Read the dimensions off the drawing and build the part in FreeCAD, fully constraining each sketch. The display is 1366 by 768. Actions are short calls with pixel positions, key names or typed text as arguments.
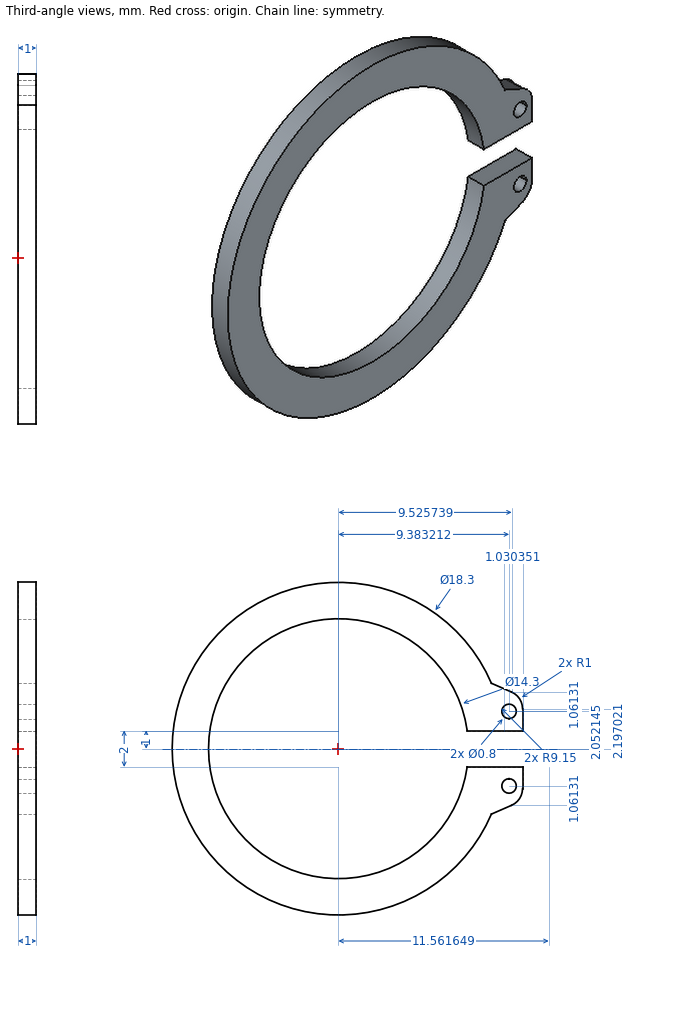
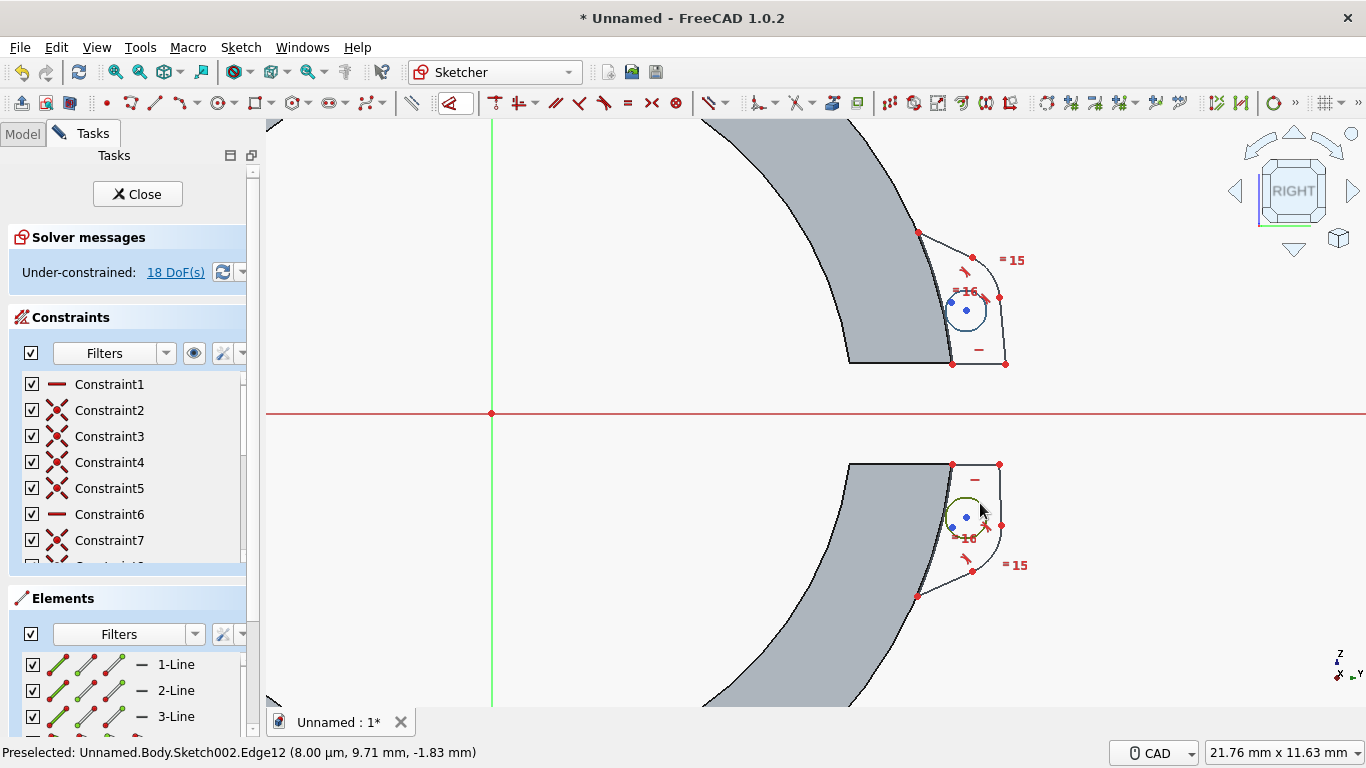
click(628, 104)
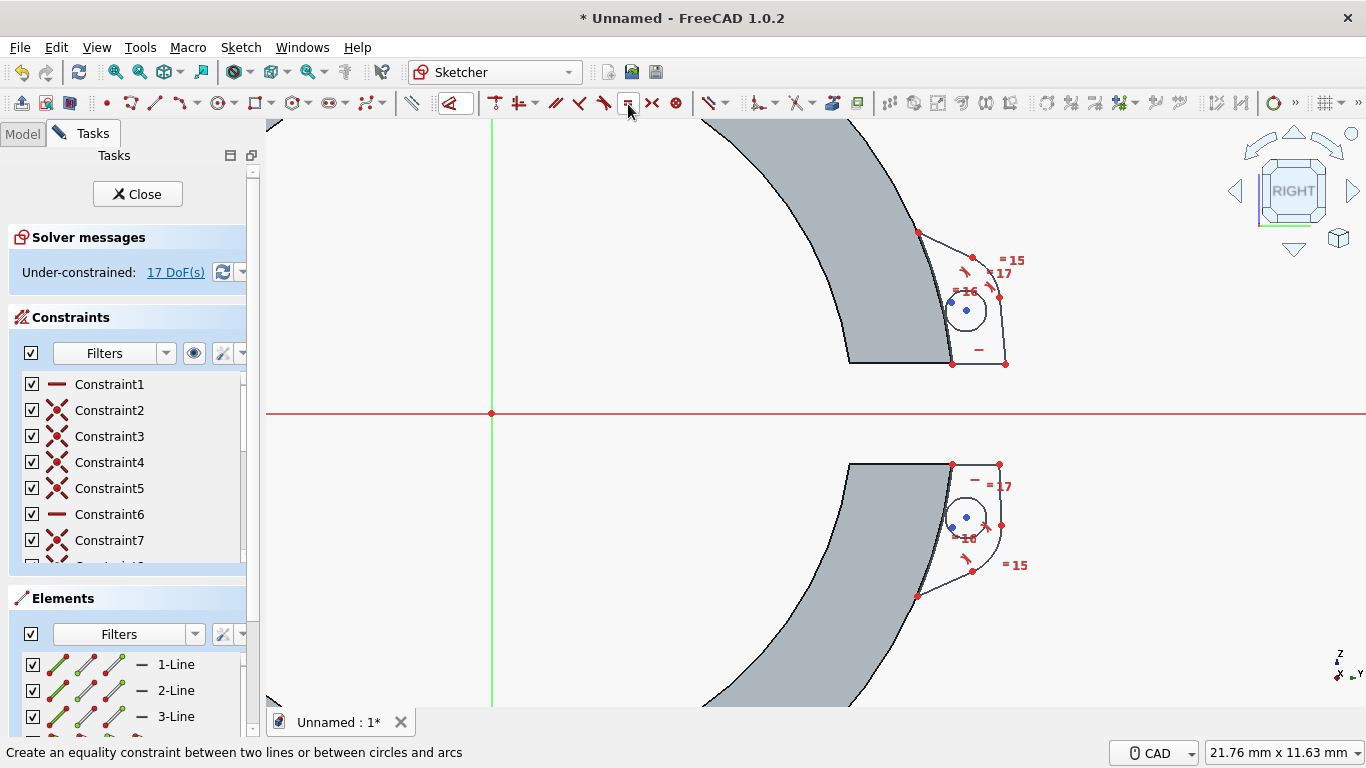
click(951, 302)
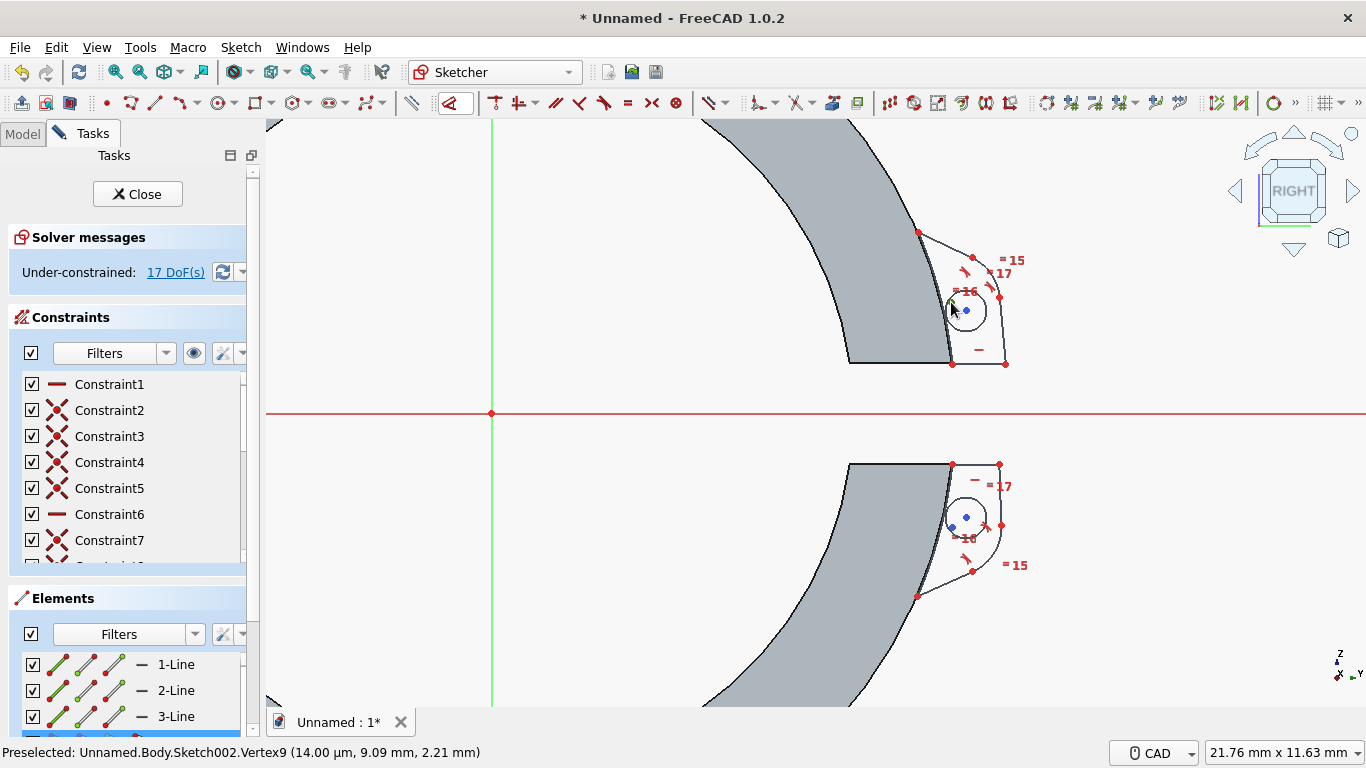
click(953, 527)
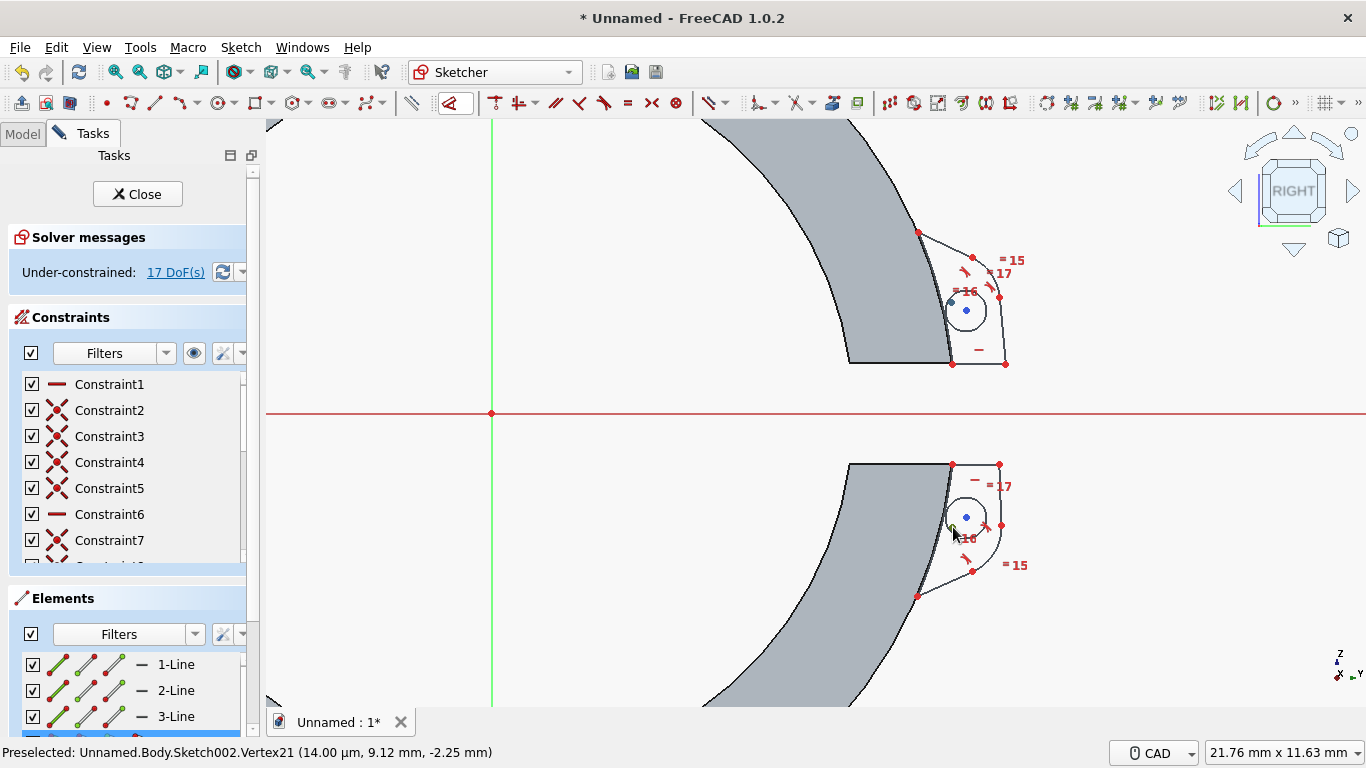
click(359, 414)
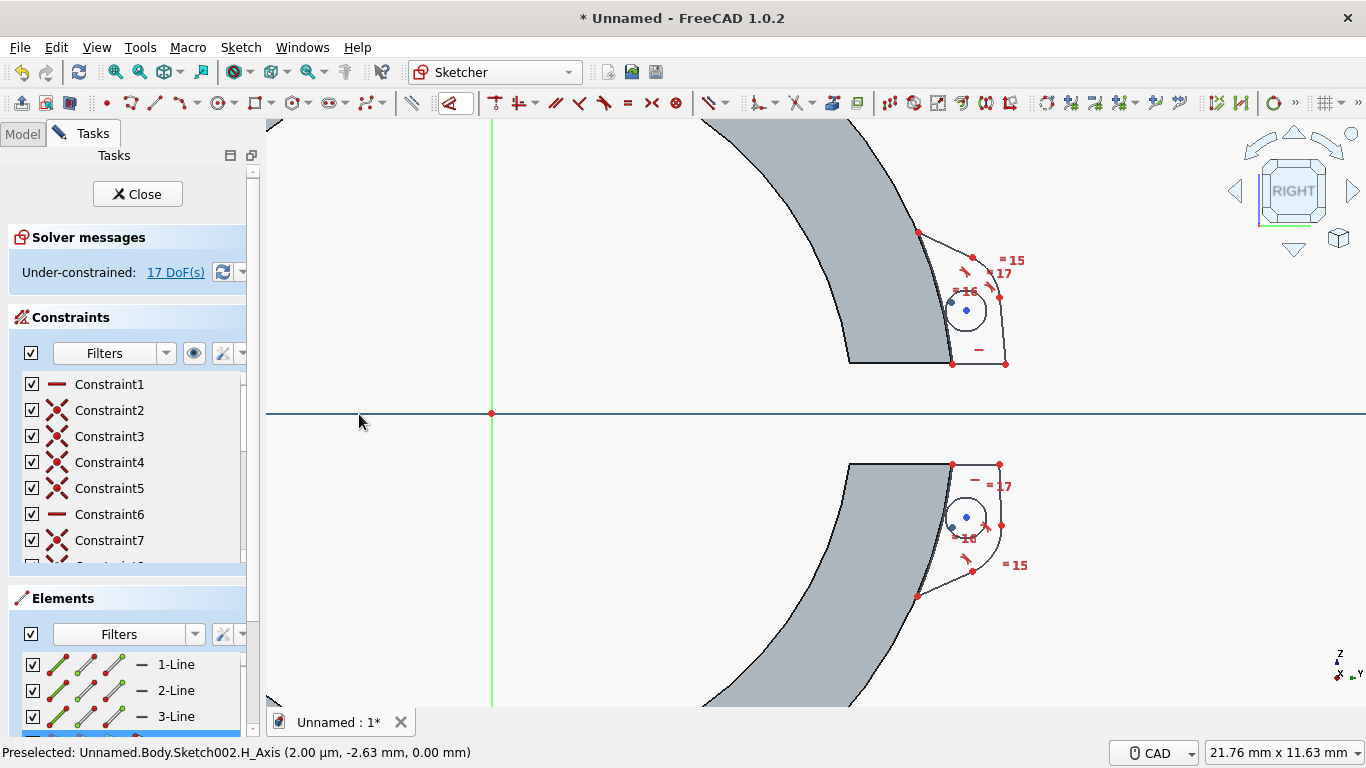
click(652, 104)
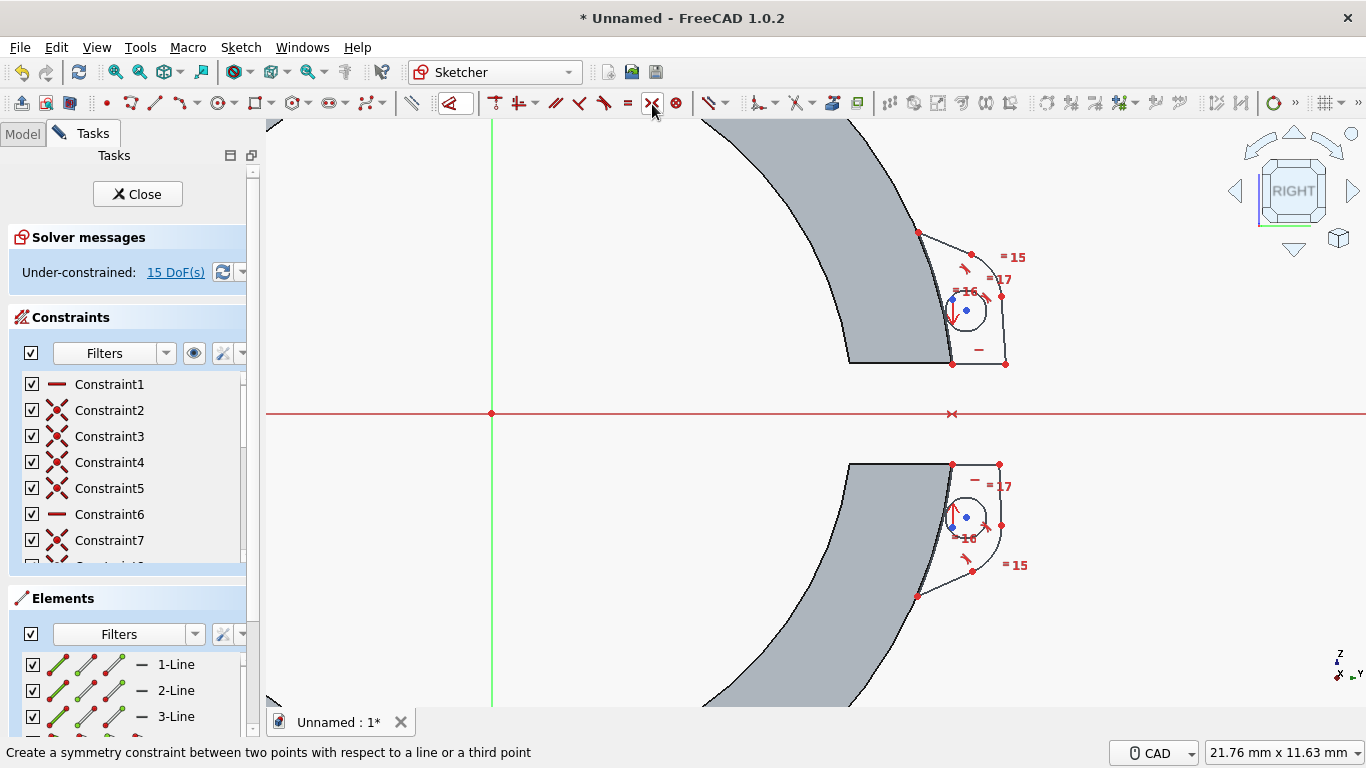
click(966, 311)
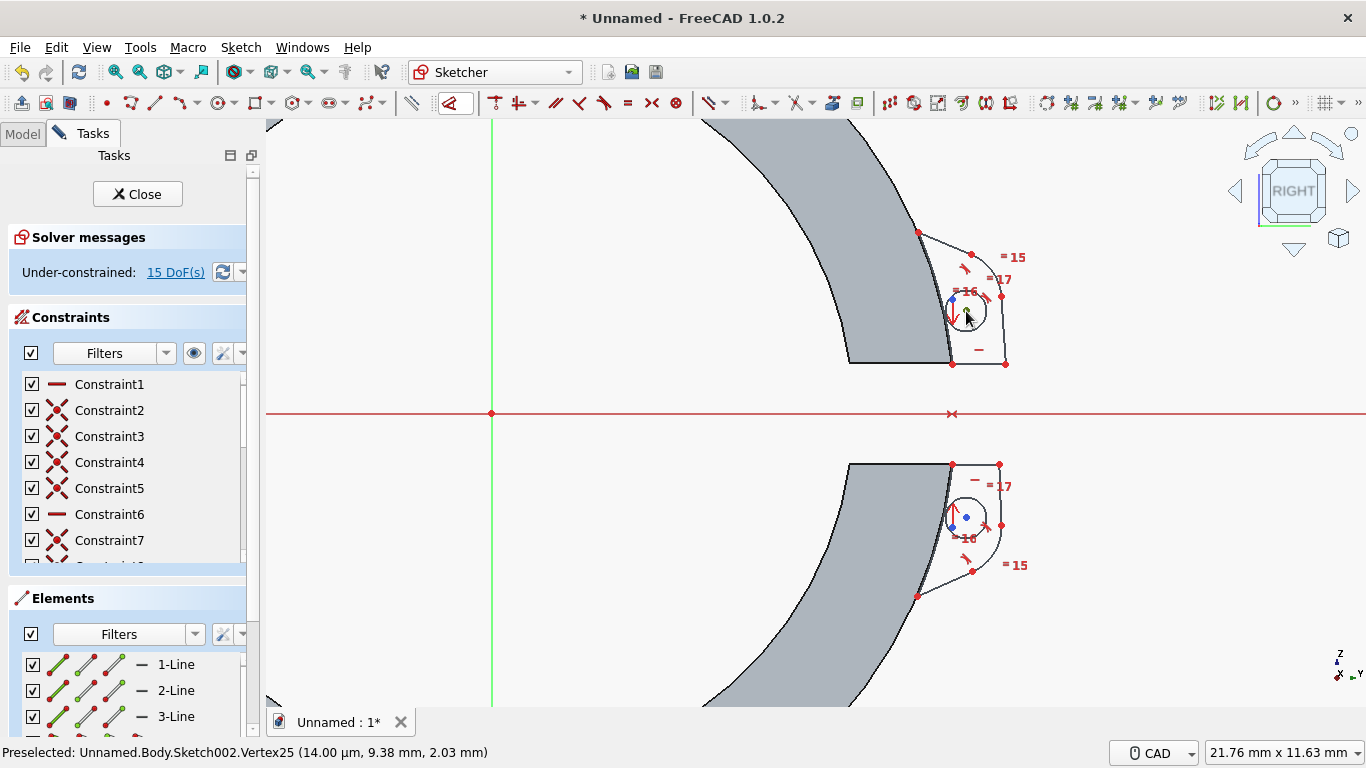
click(966, 518)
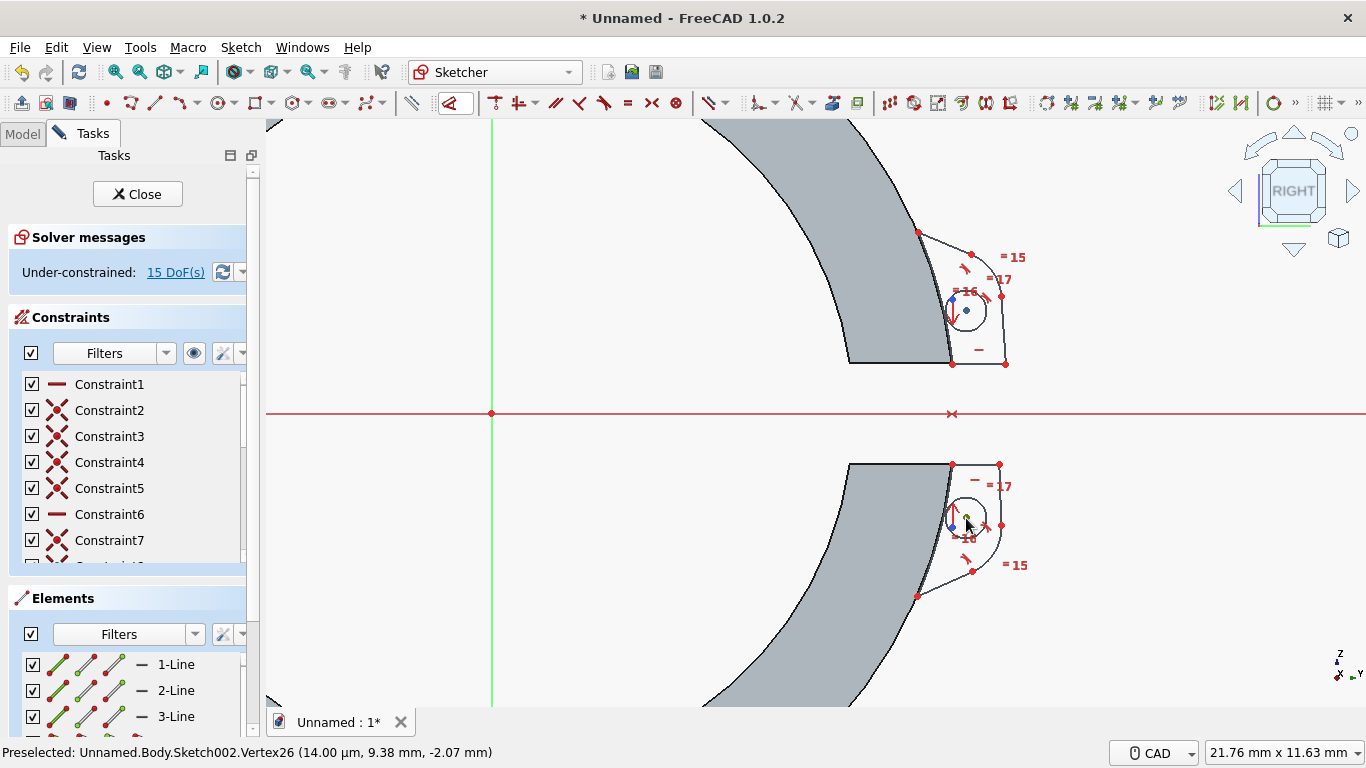
click(359, 414)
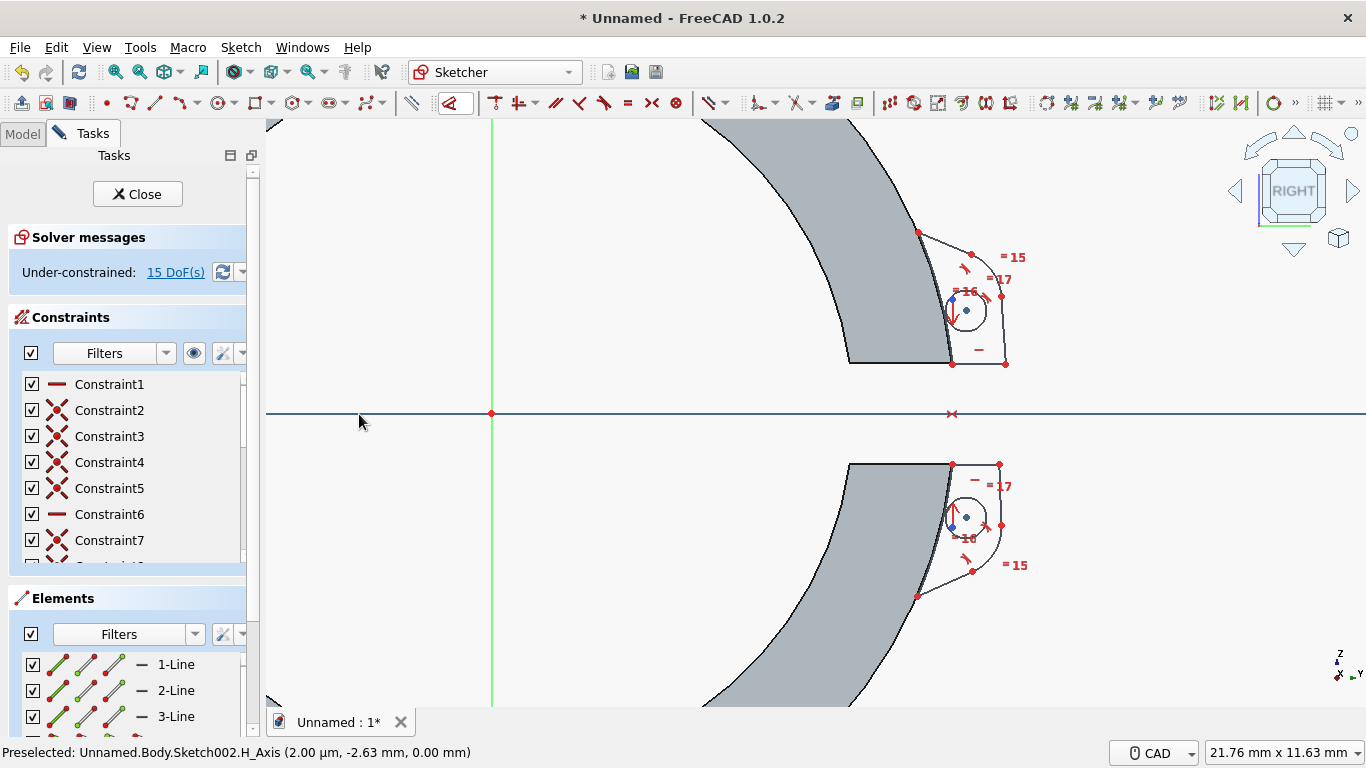
click(652, 104)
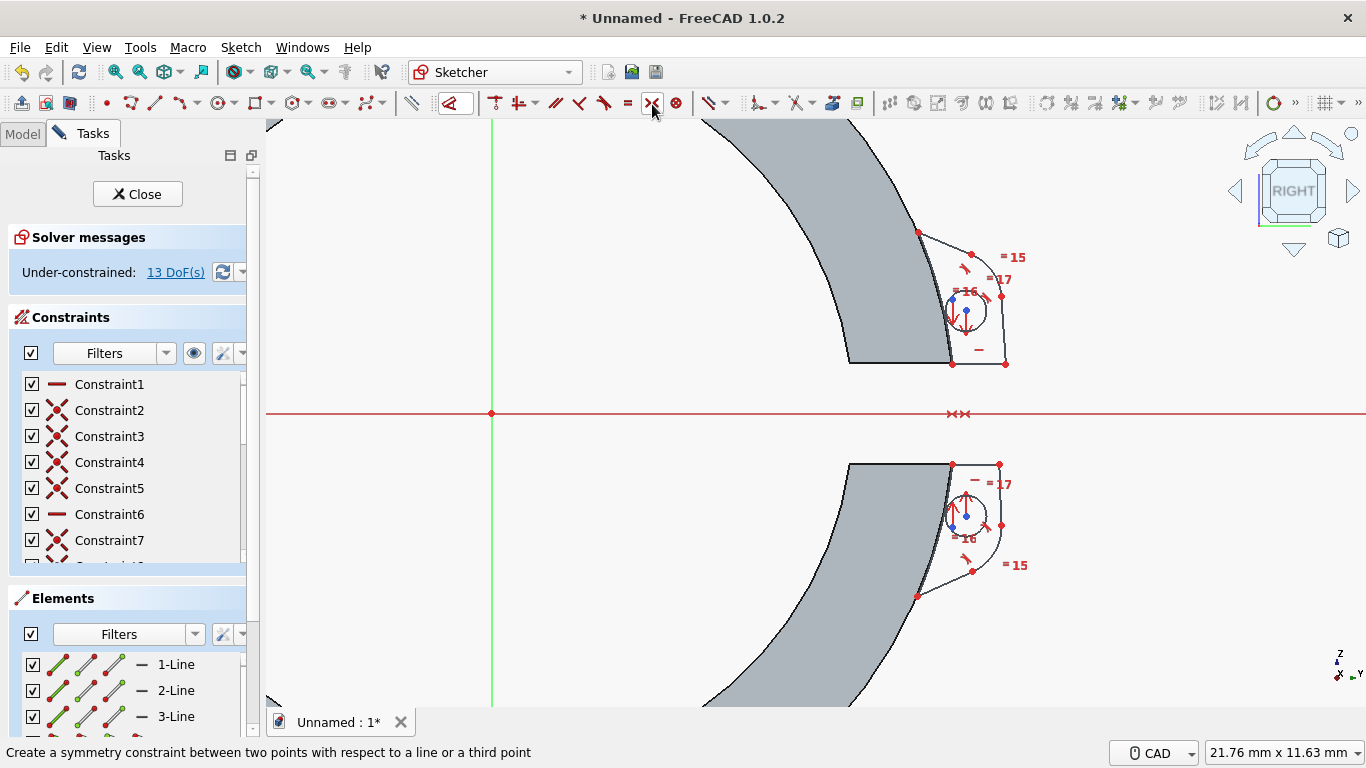
click(1006, 364)